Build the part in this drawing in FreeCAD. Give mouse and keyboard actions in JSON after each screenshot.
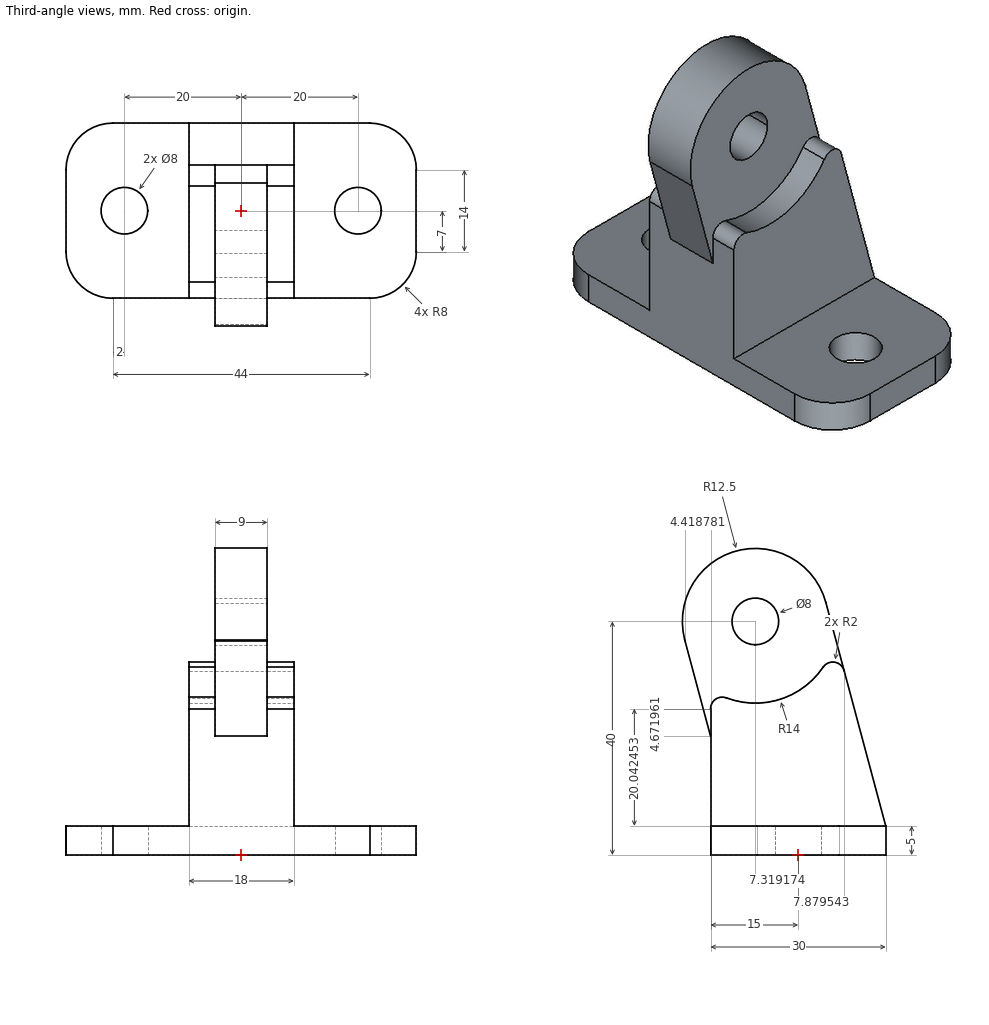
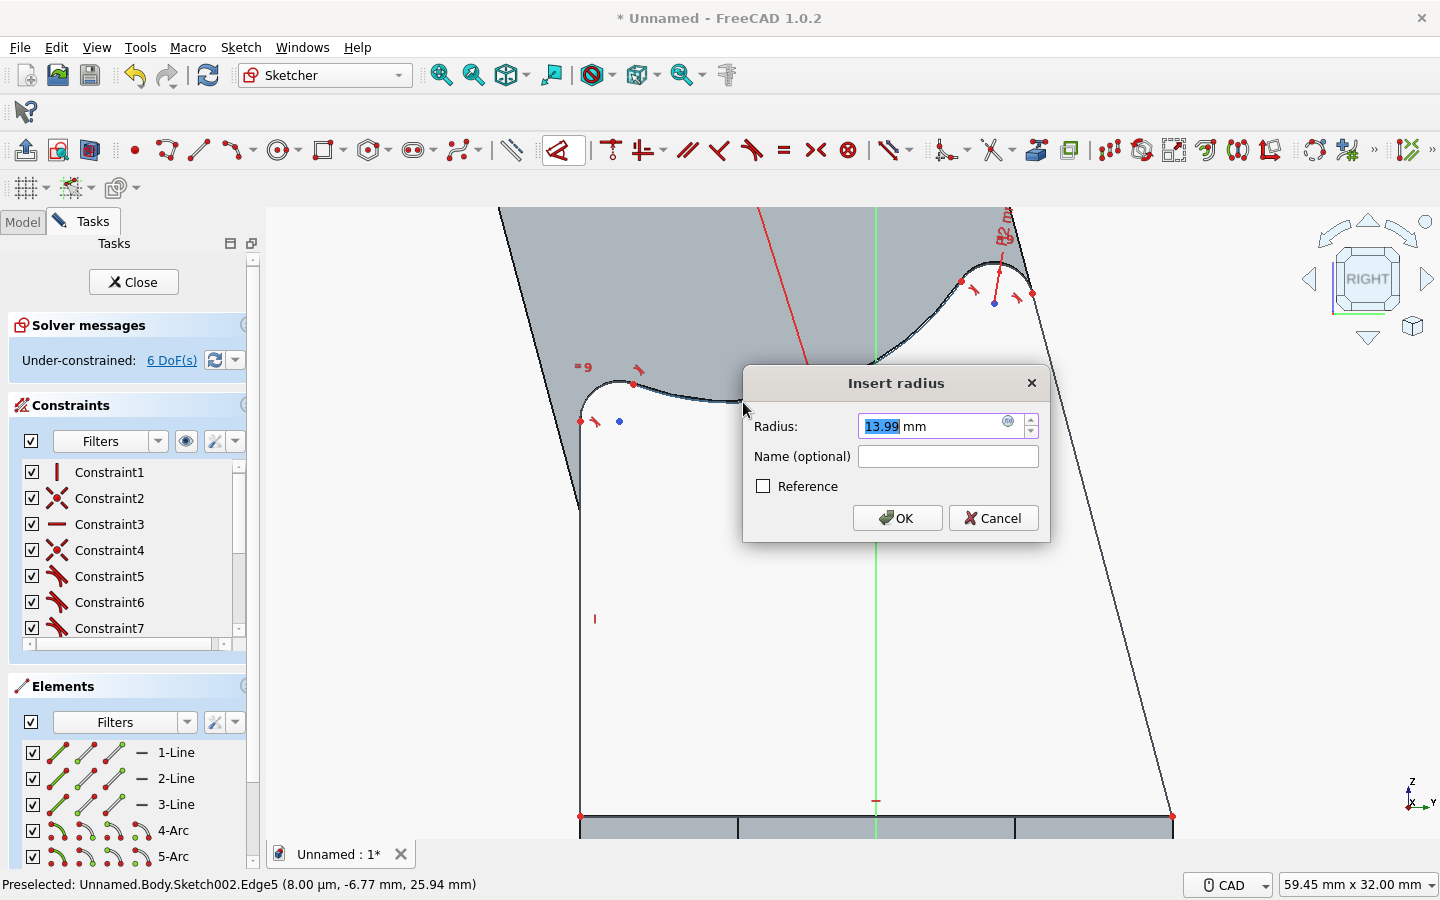
{"action": "type", "text": "14"}
{"action": "key", "text": "Return"}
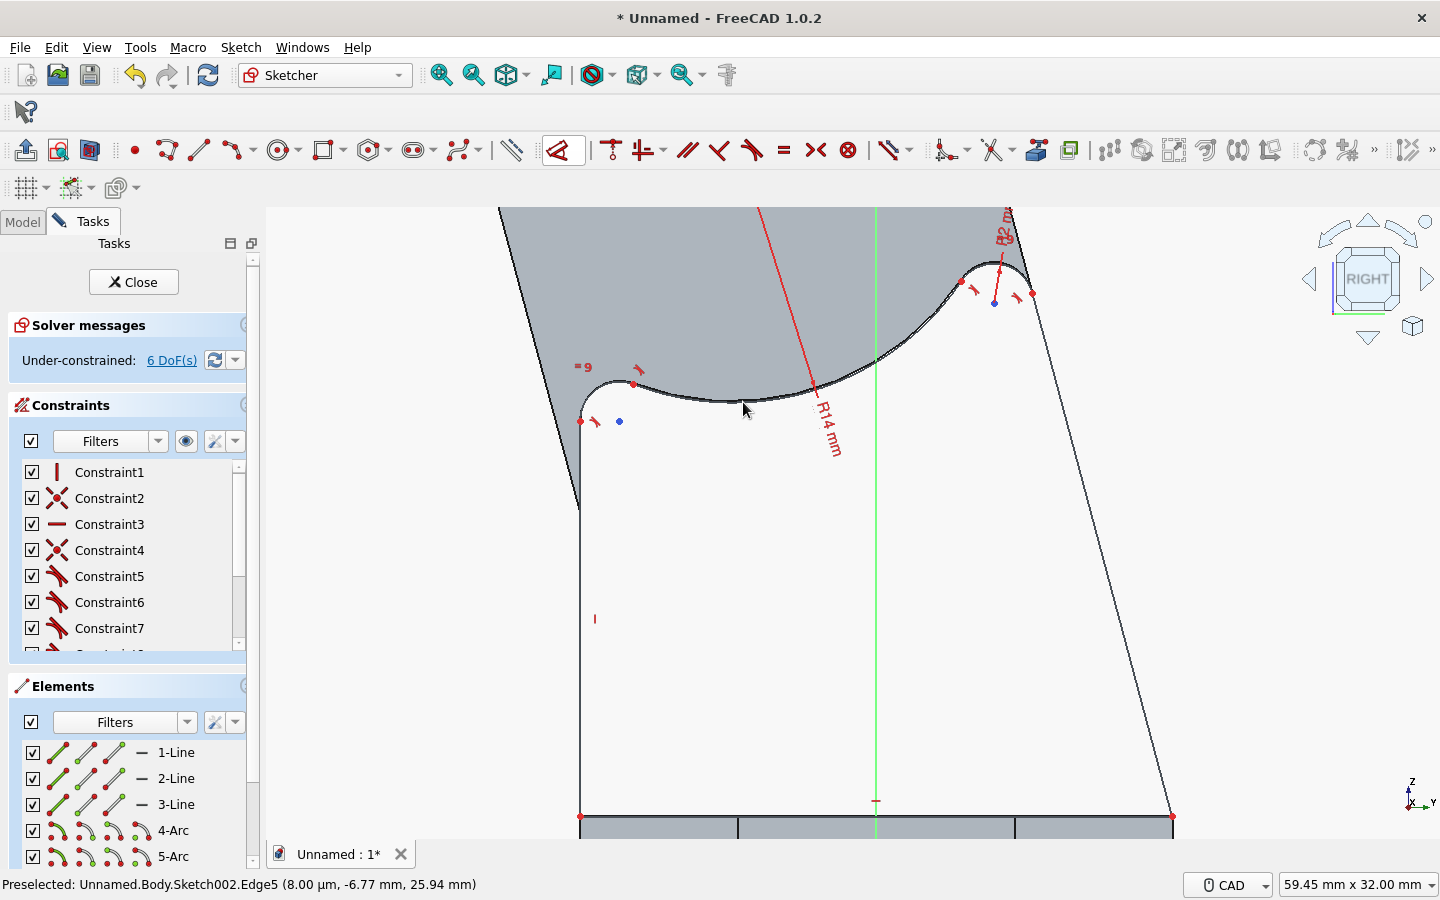
{"action": "scroll", "coordinate": [598, 390], "scroll_direction": "down", "scroll_amount": 2}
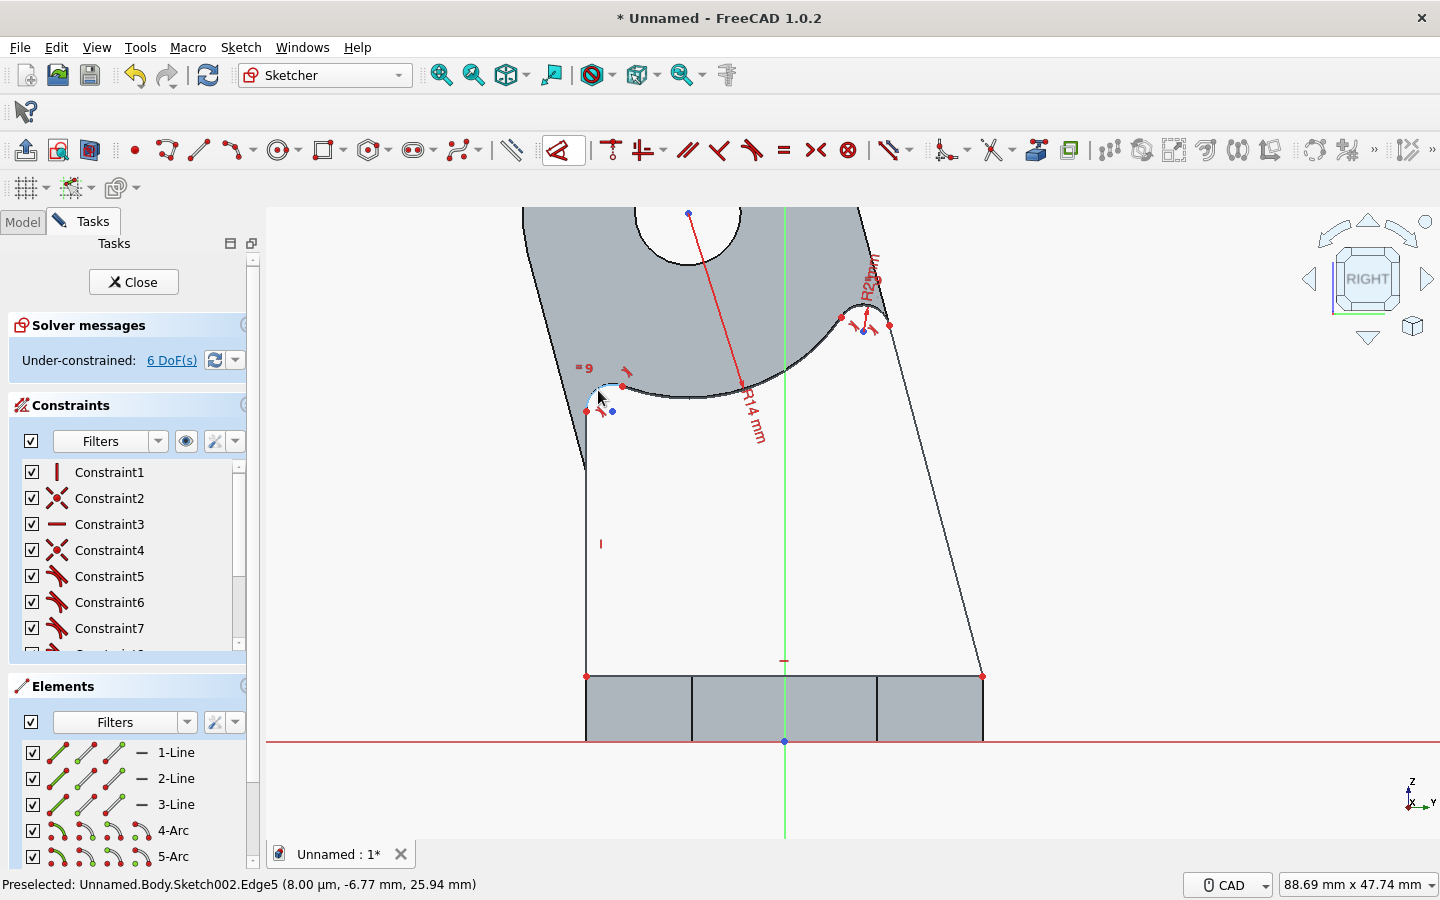
{"action": "left_click", "coordinate": [705, 676]}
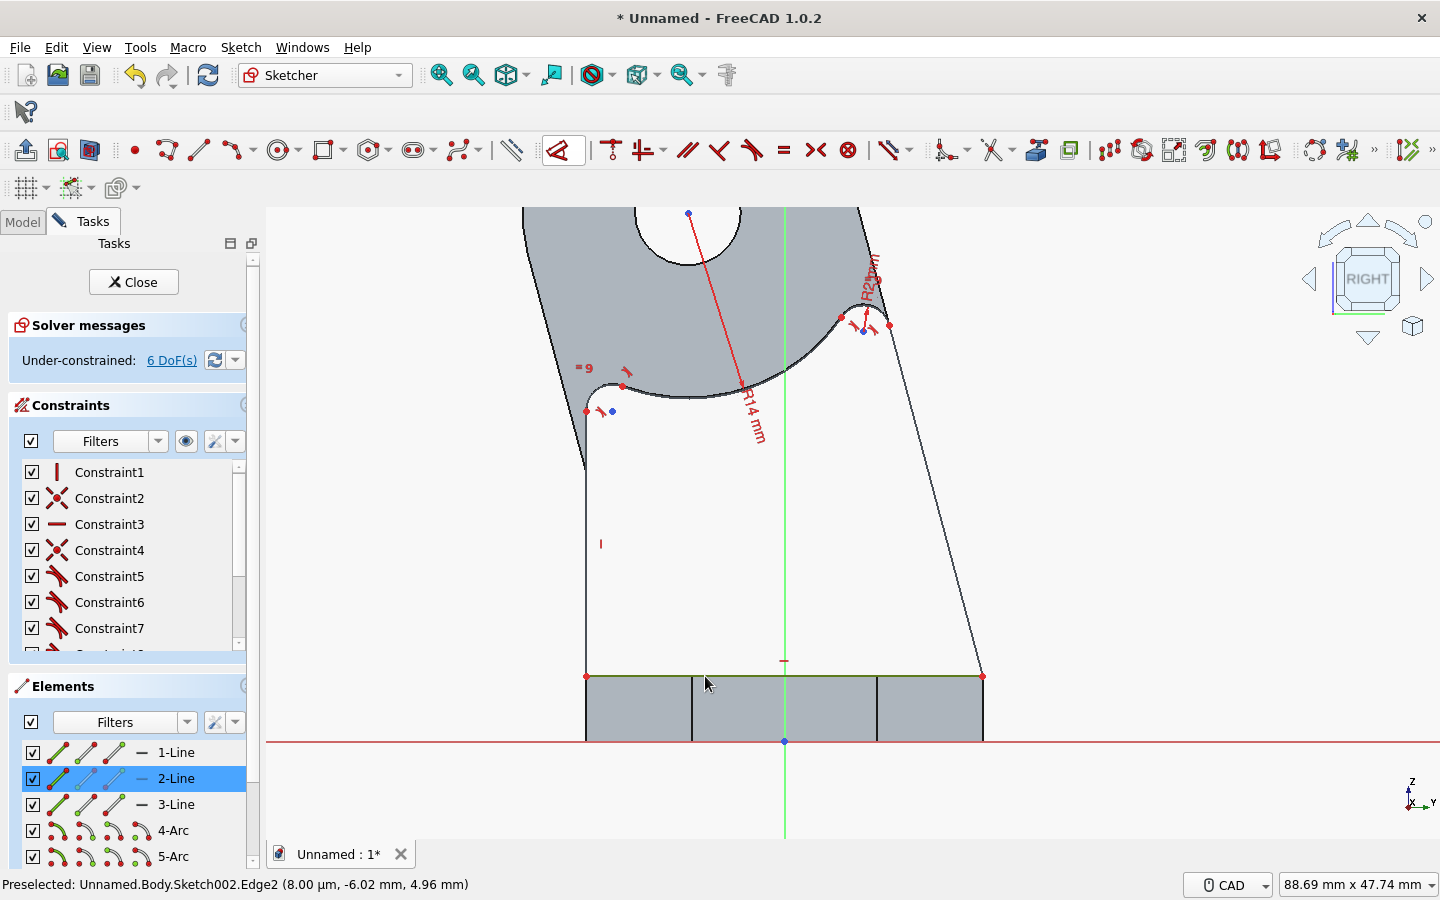
{"action": "key", "text": "l"}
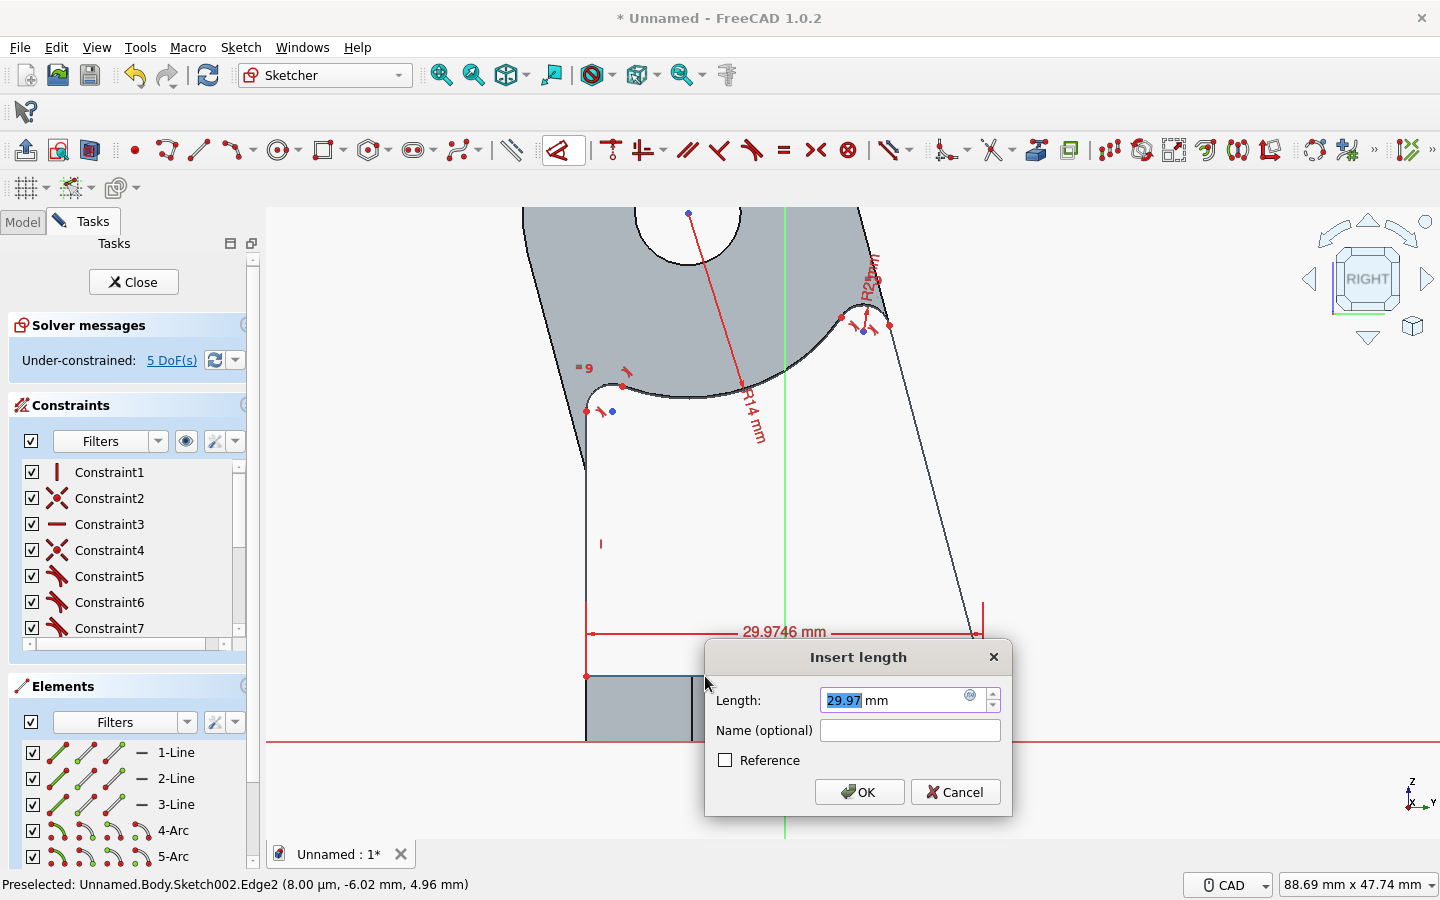
{"action": "type", "text": "30"}
{"action": "key", "text": "Return"}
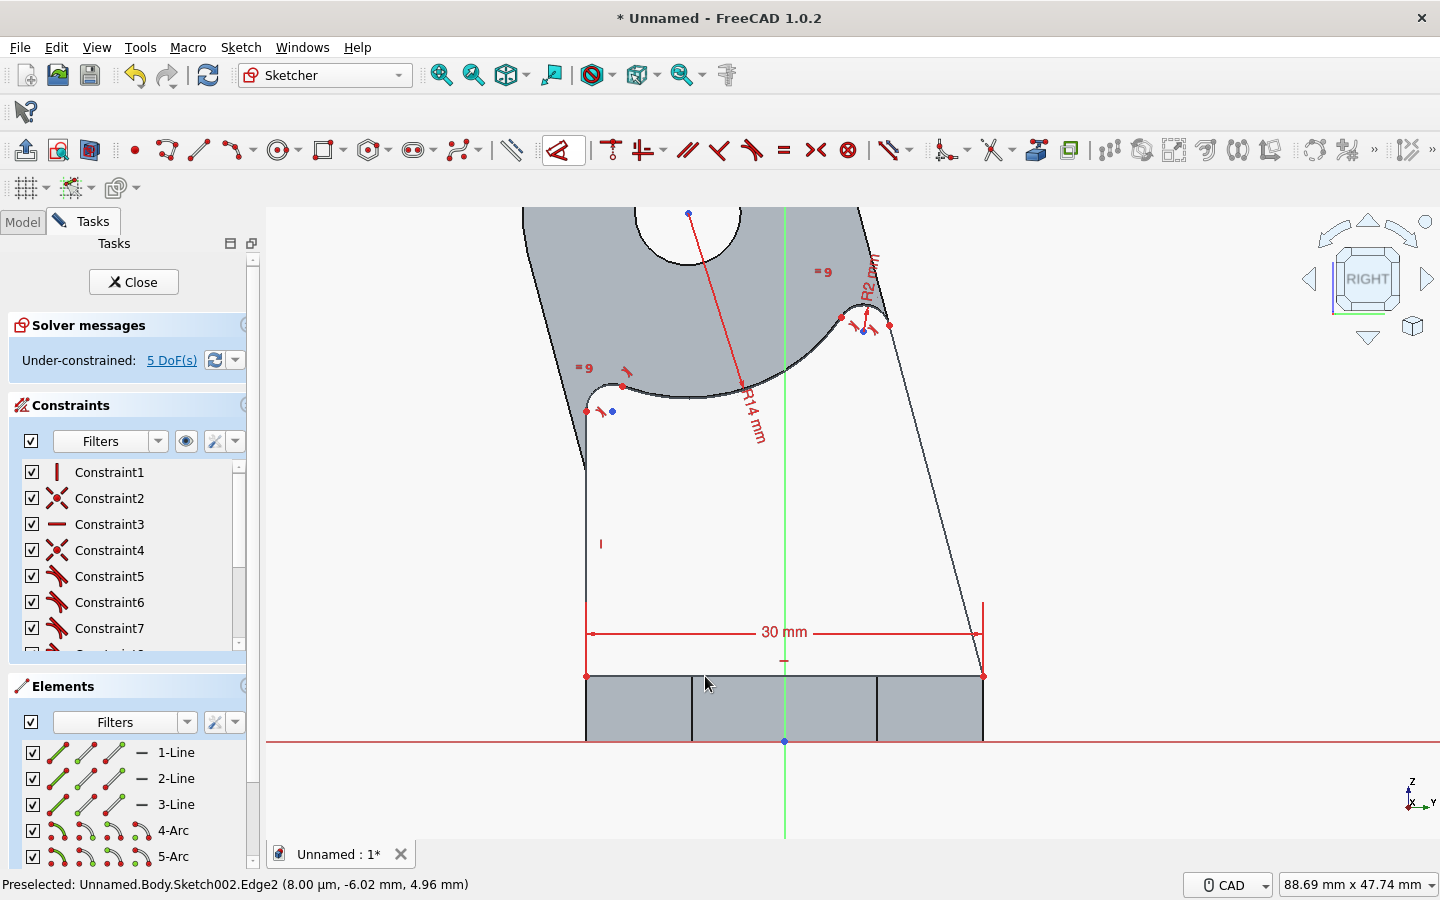
{"action": "left_click", "coordinate": [586, 676]}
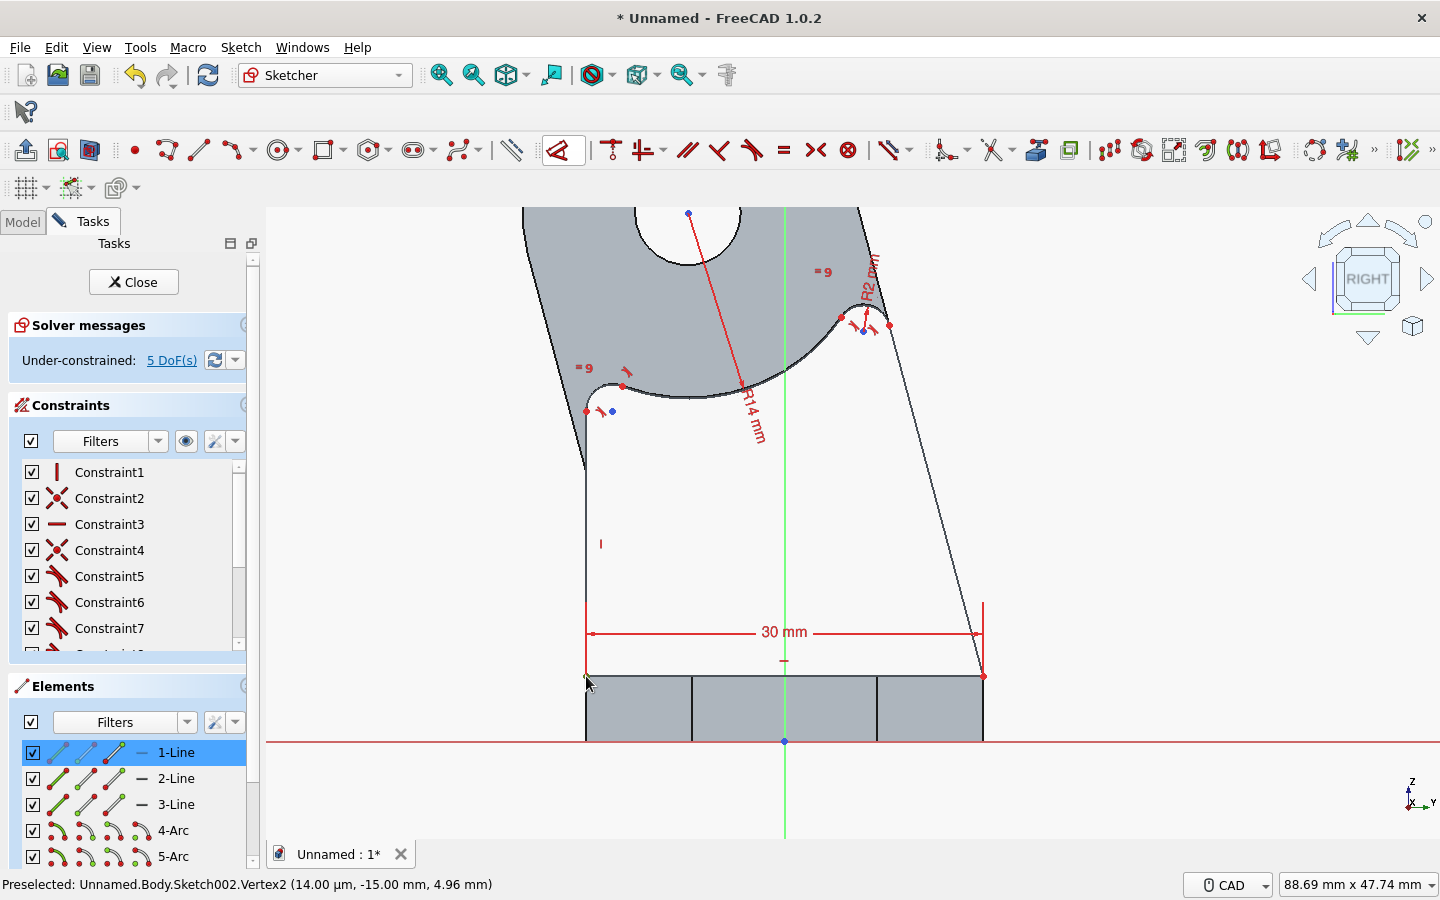
{"action": "key", "text": "i"}